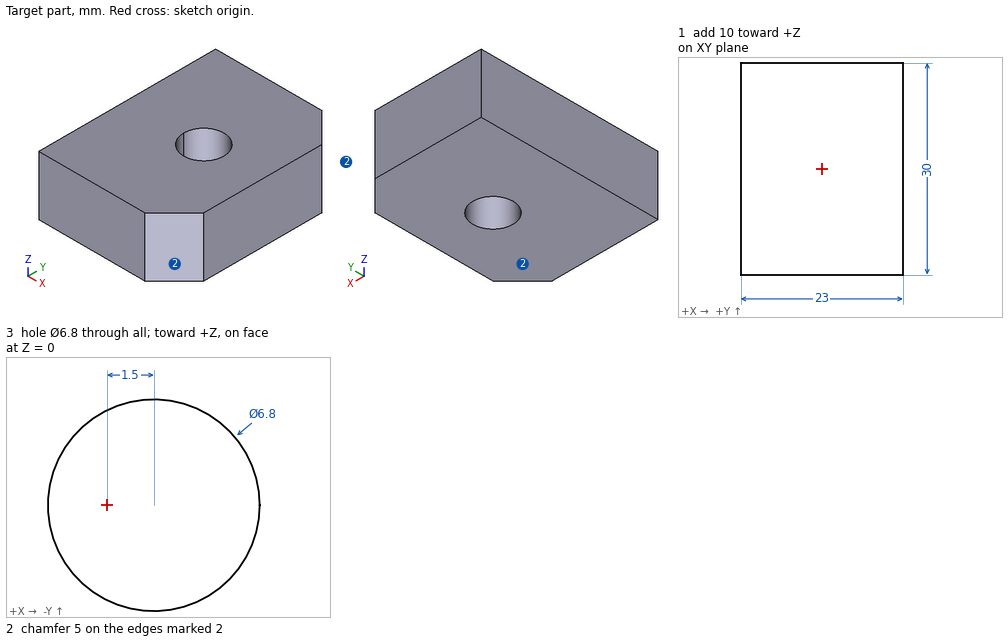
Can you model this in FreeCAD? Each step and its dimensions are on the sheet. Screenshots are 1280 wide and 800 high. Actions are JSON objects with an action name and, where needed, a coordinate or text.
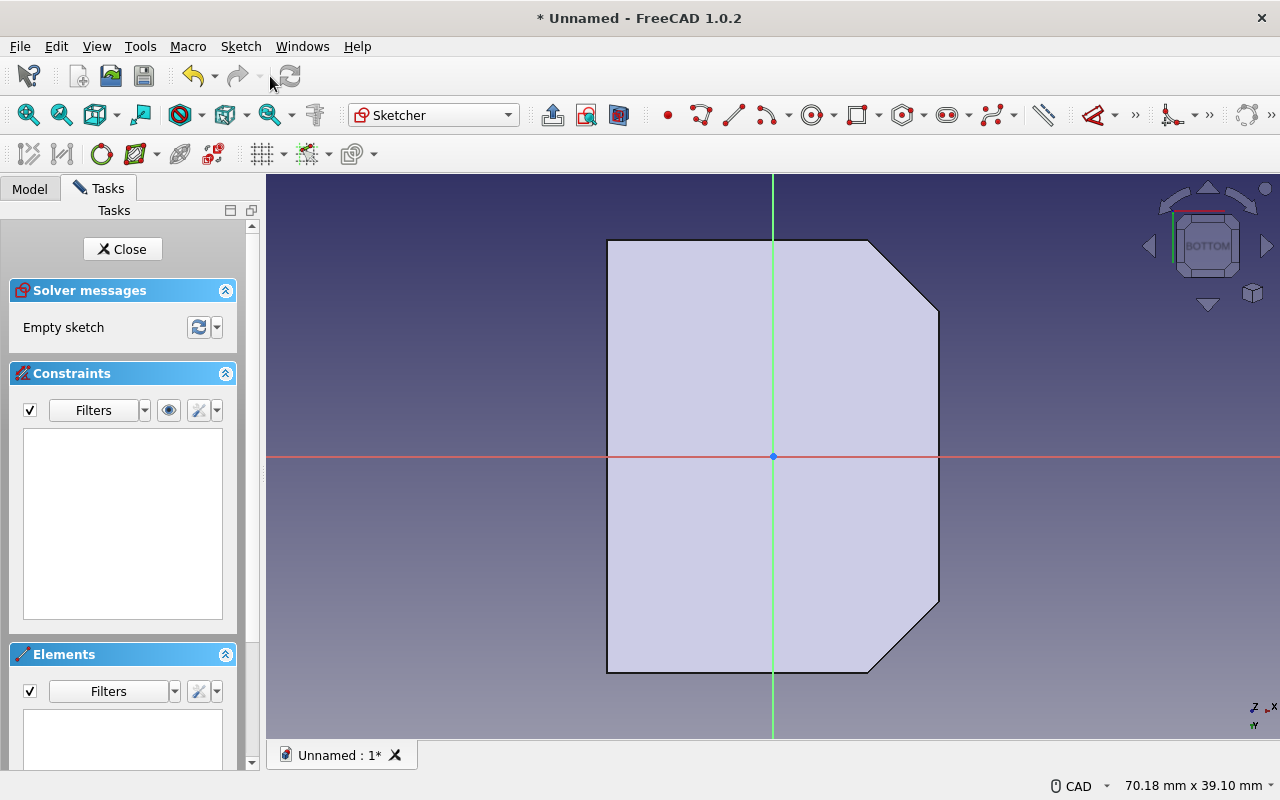
{"action": "scroll", "coordinate": [834, 456], "scroll_direction": "up", "scroll_amount": 6}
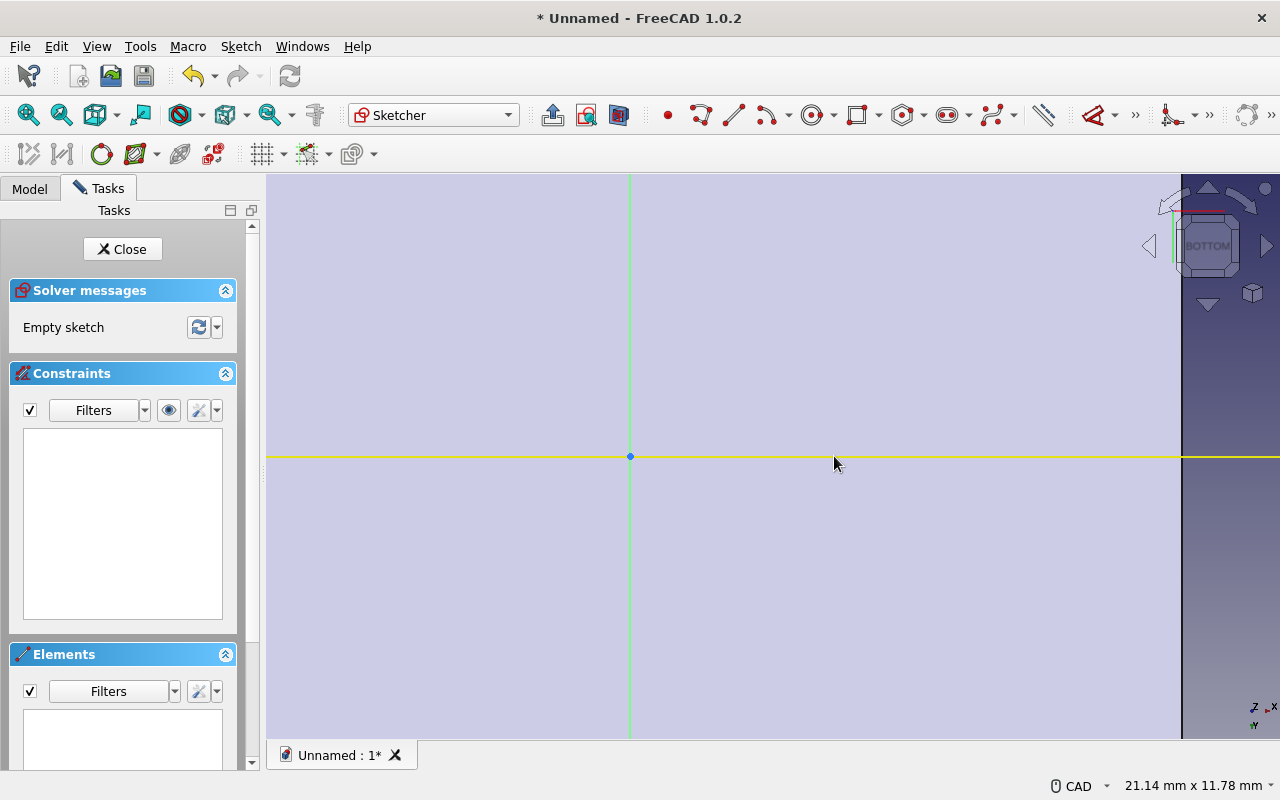
{"action": "left_click", "coordinate": [812, 116]}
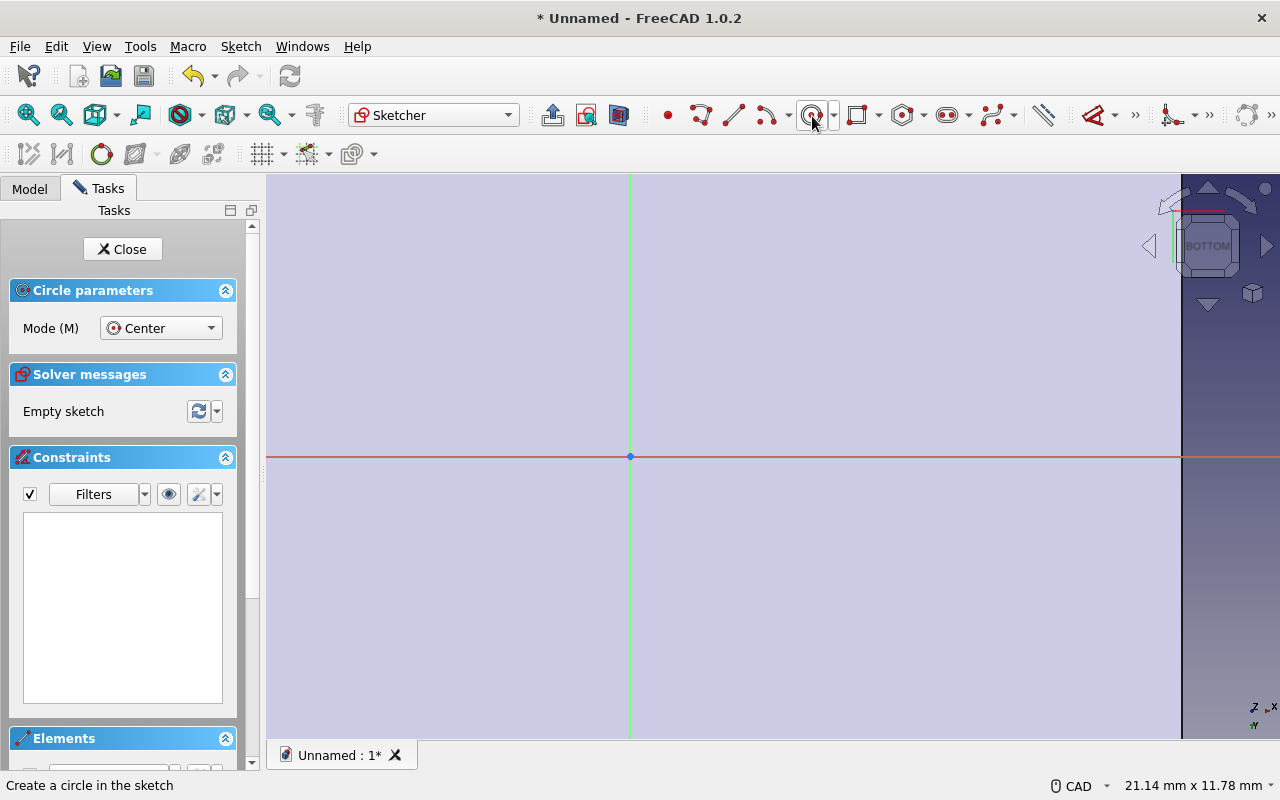
{"action": "left_click", "coordinate": [702, 456]}
{"action": "left_click", "coordinate": [817, 341]}
{"action": "key", "text": "Escape"}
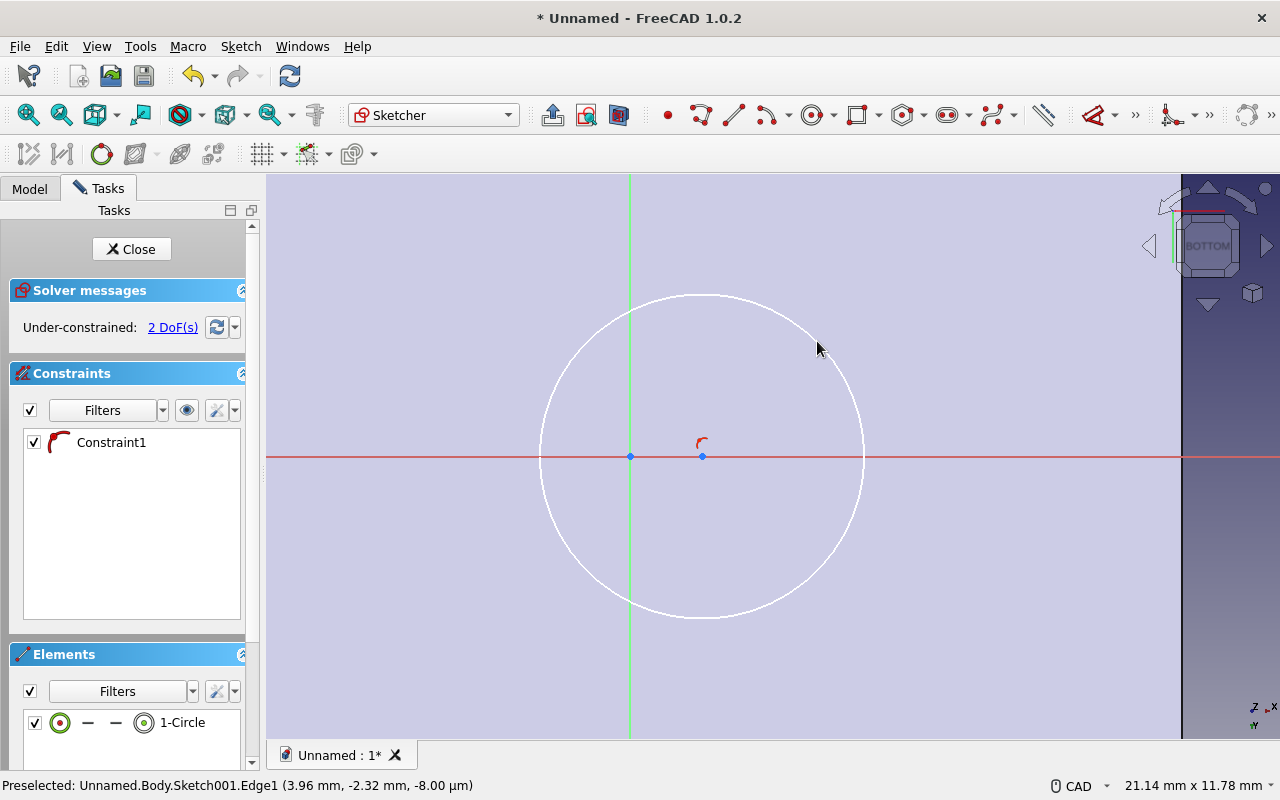
{"action": "left_click", "coordinate": [1092, 116]}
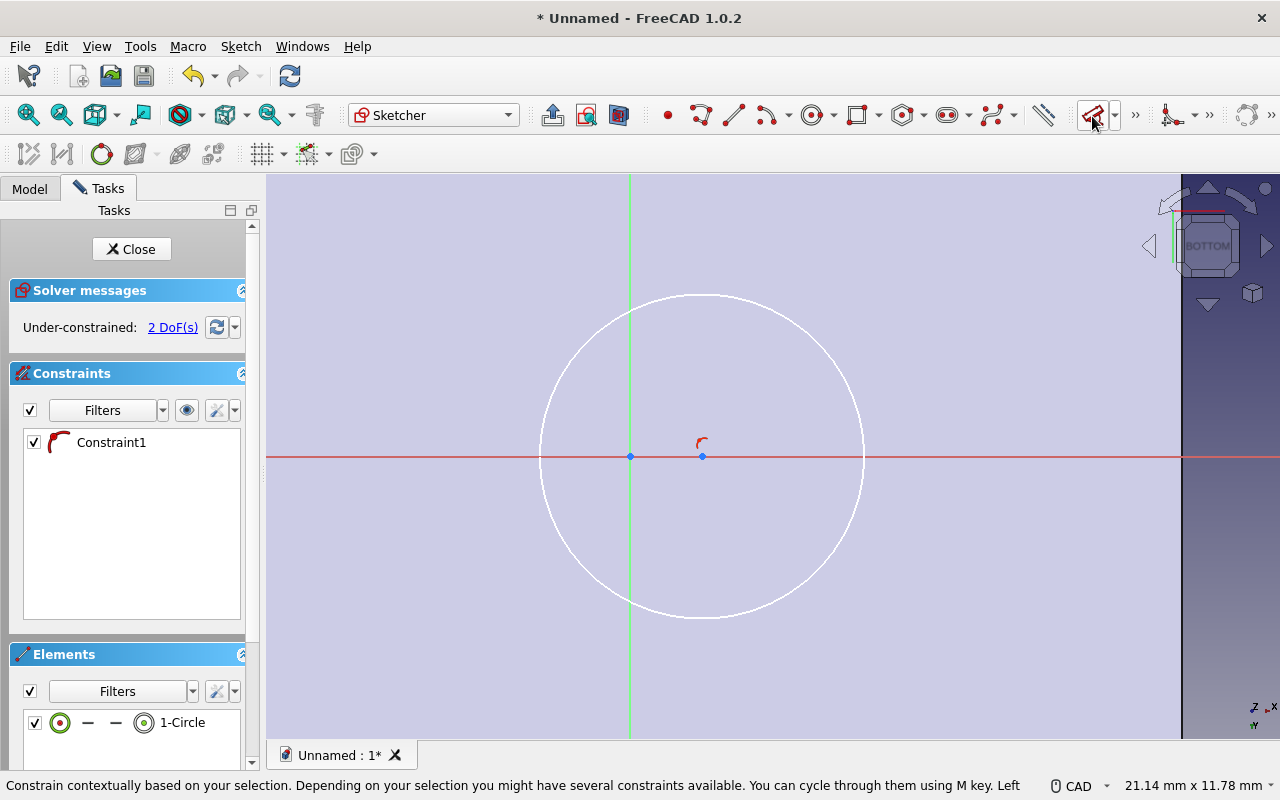
{"action": "left_click", "coordinate": [816, 341]}
{"action": "left_click", "coordinate": [838, 318]}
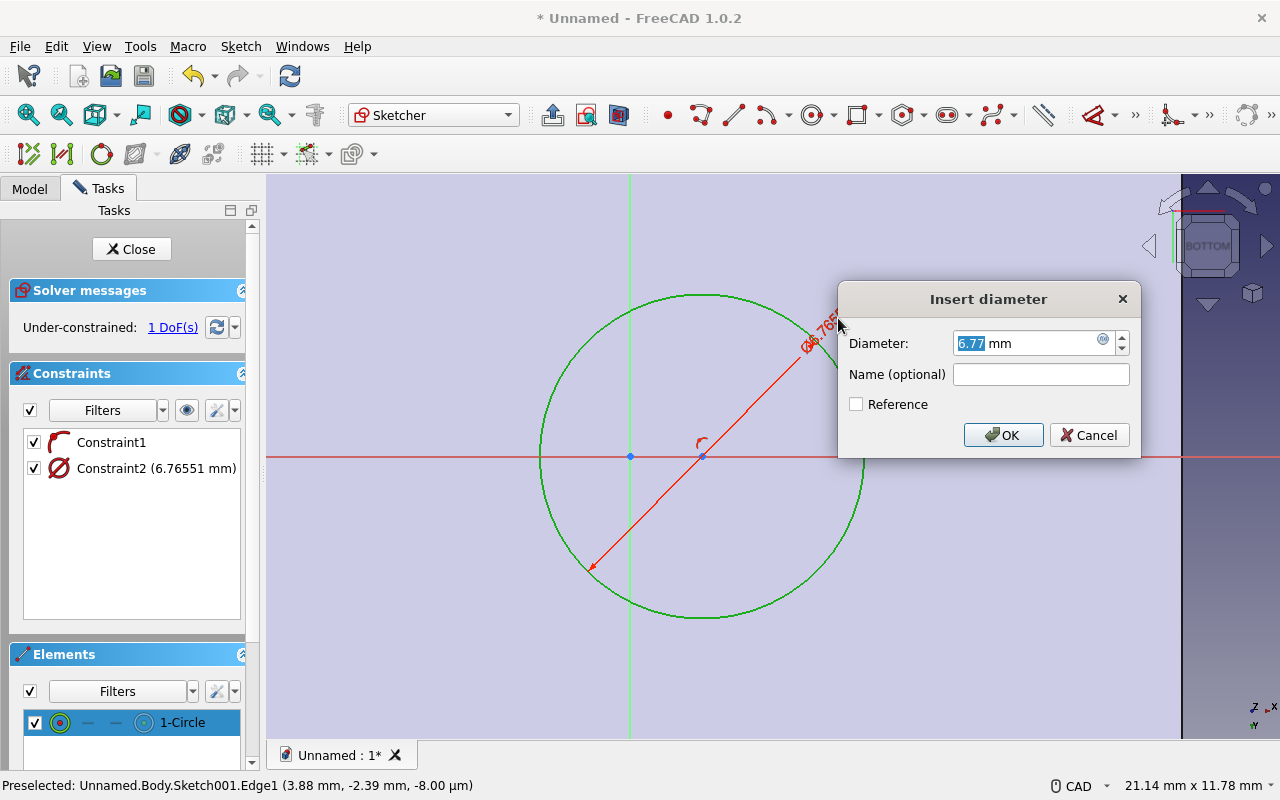
{"action": "type", "text": "6.8"}
{"action": "key", "text": "Return"}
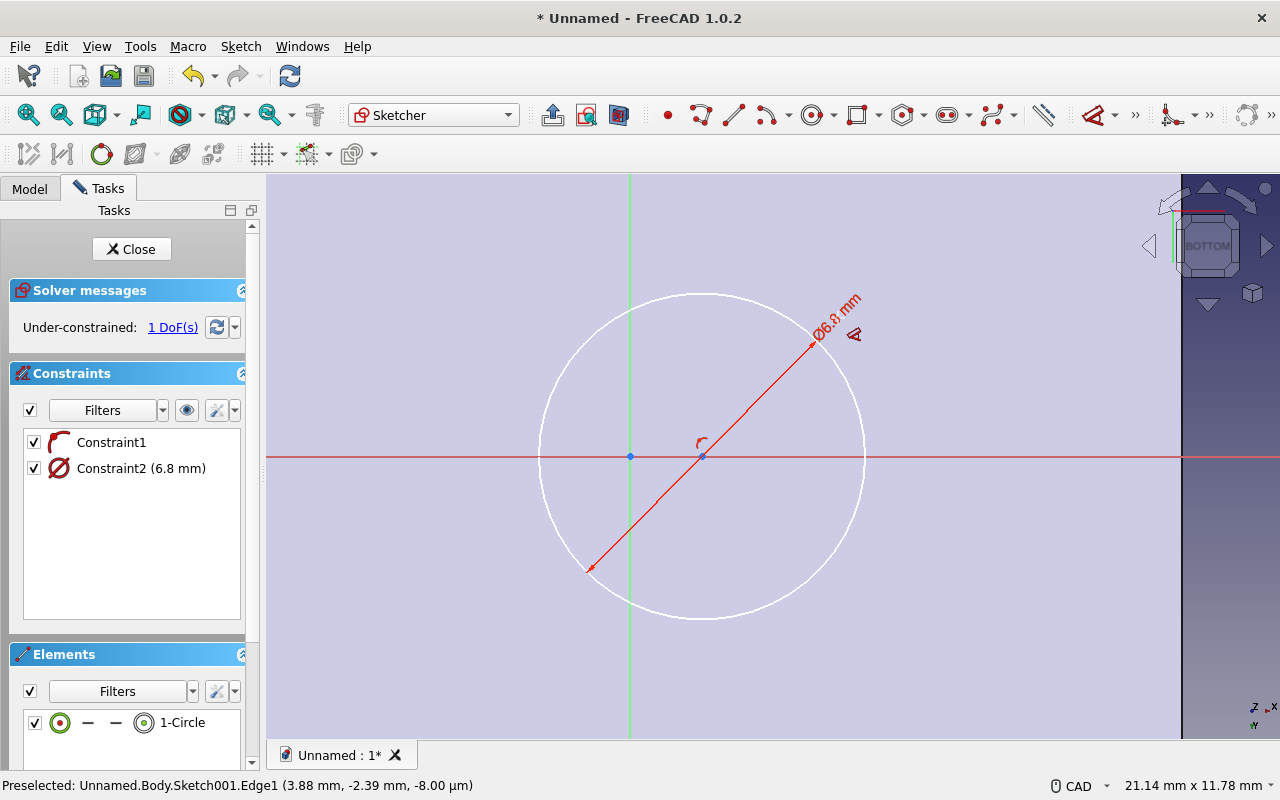
{"action": "left_click", "coordinate": [702, 456]}
{"action": "left_click", "coordinate": [666, 490]}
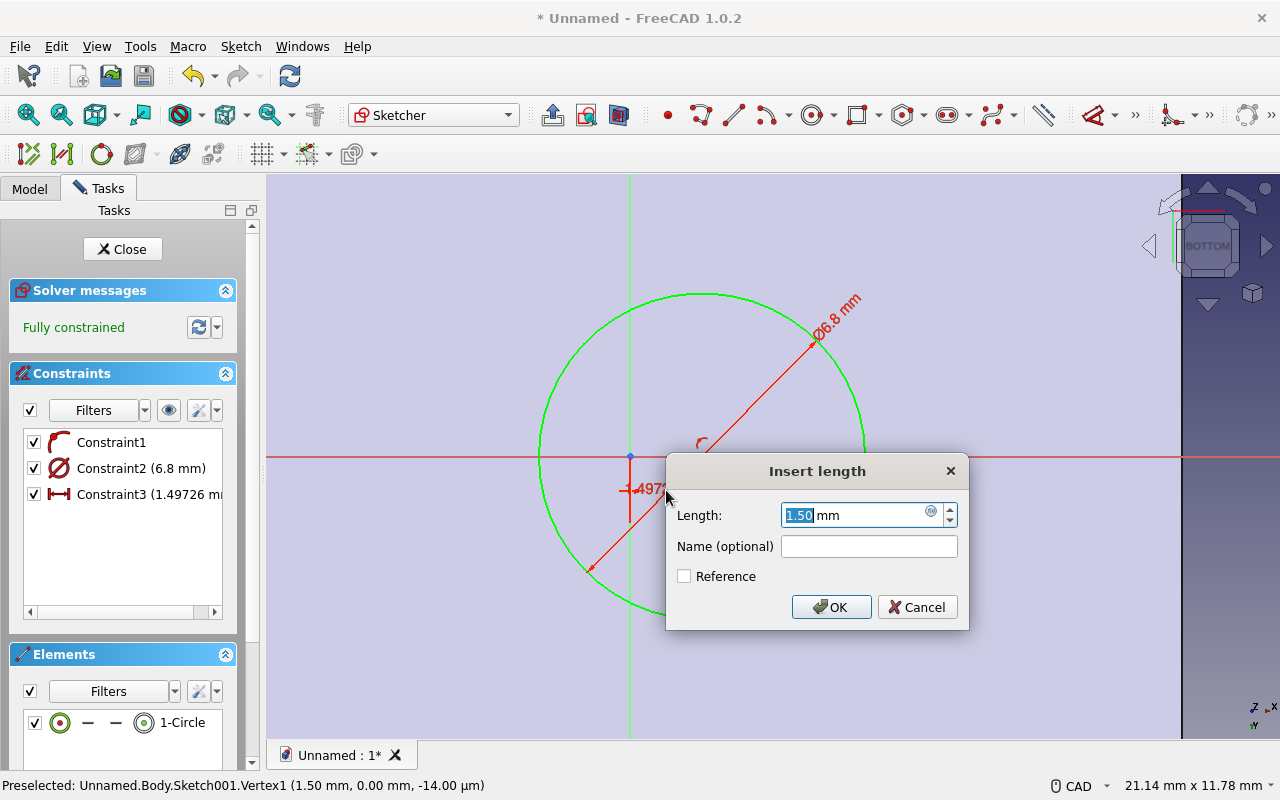
{"action": "type", "text": "1.5"}
{"action": "key", "text": "Return"}
{"action": "key", "text": "Escape"}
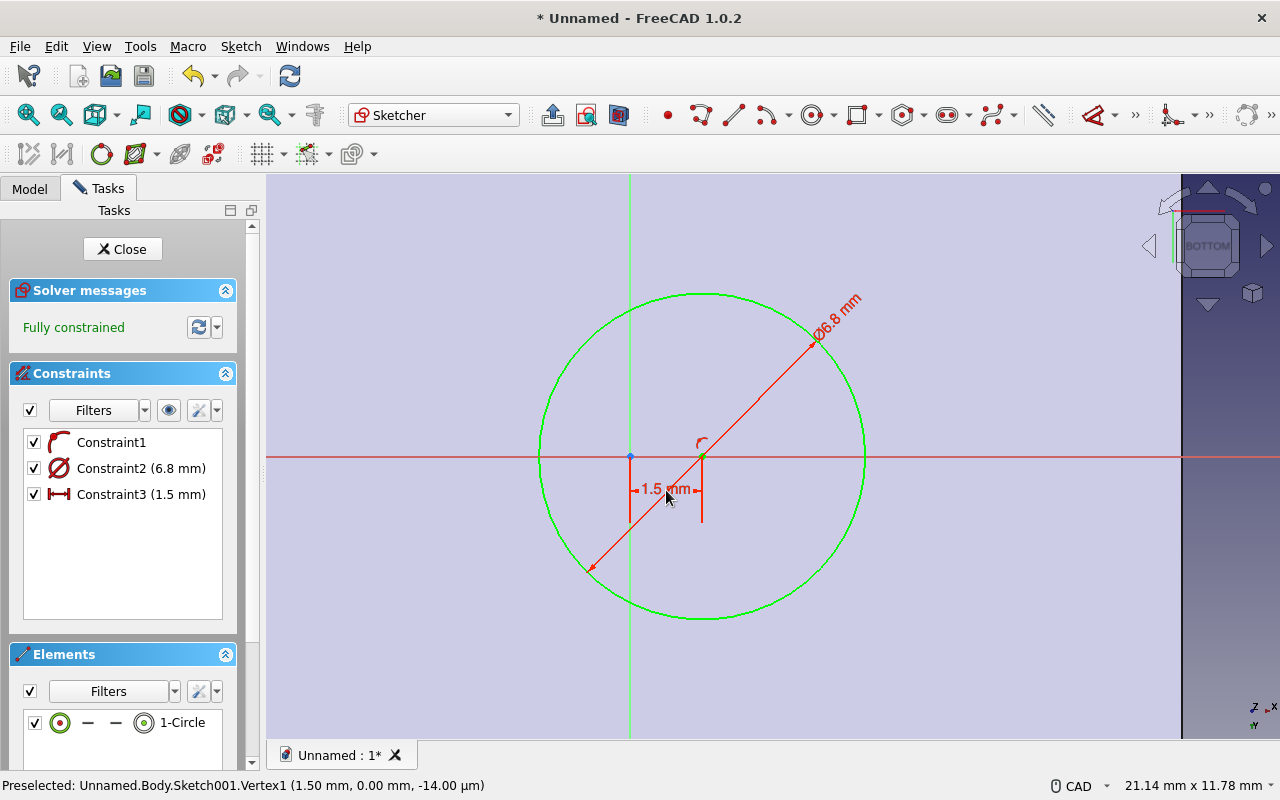
{"action": "left_click", "coordinate": [123, 249]}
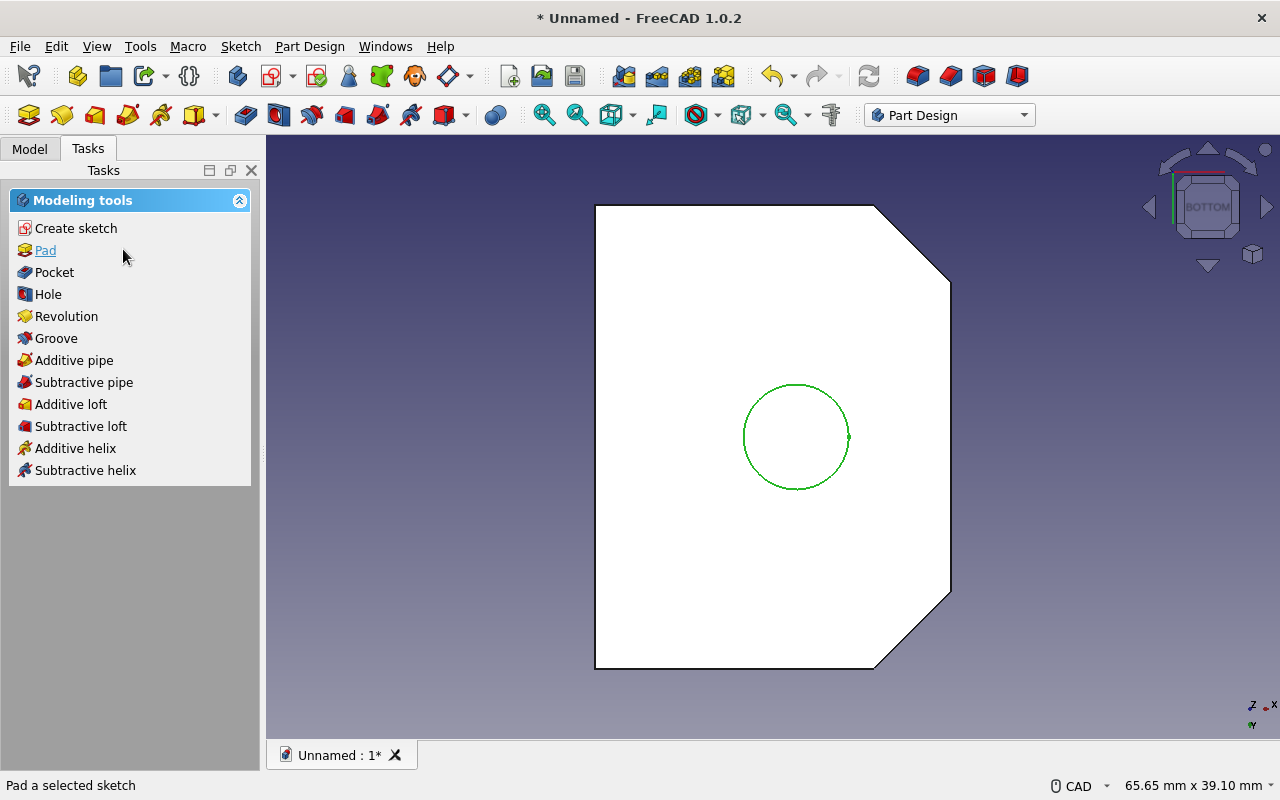
{"action": "left_click", "coordinate": [279, 116]}